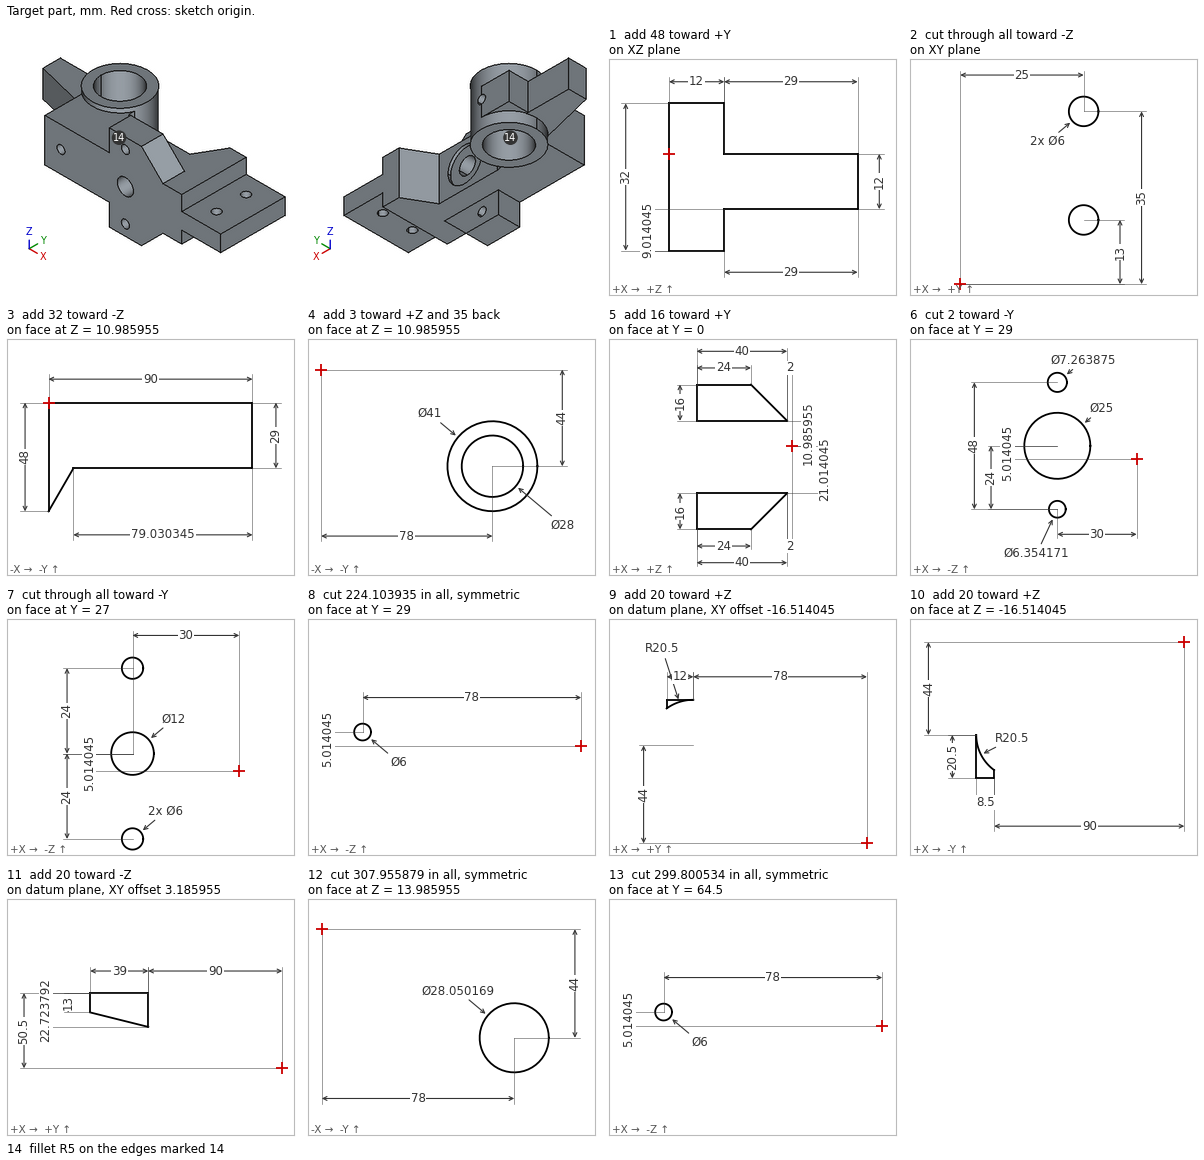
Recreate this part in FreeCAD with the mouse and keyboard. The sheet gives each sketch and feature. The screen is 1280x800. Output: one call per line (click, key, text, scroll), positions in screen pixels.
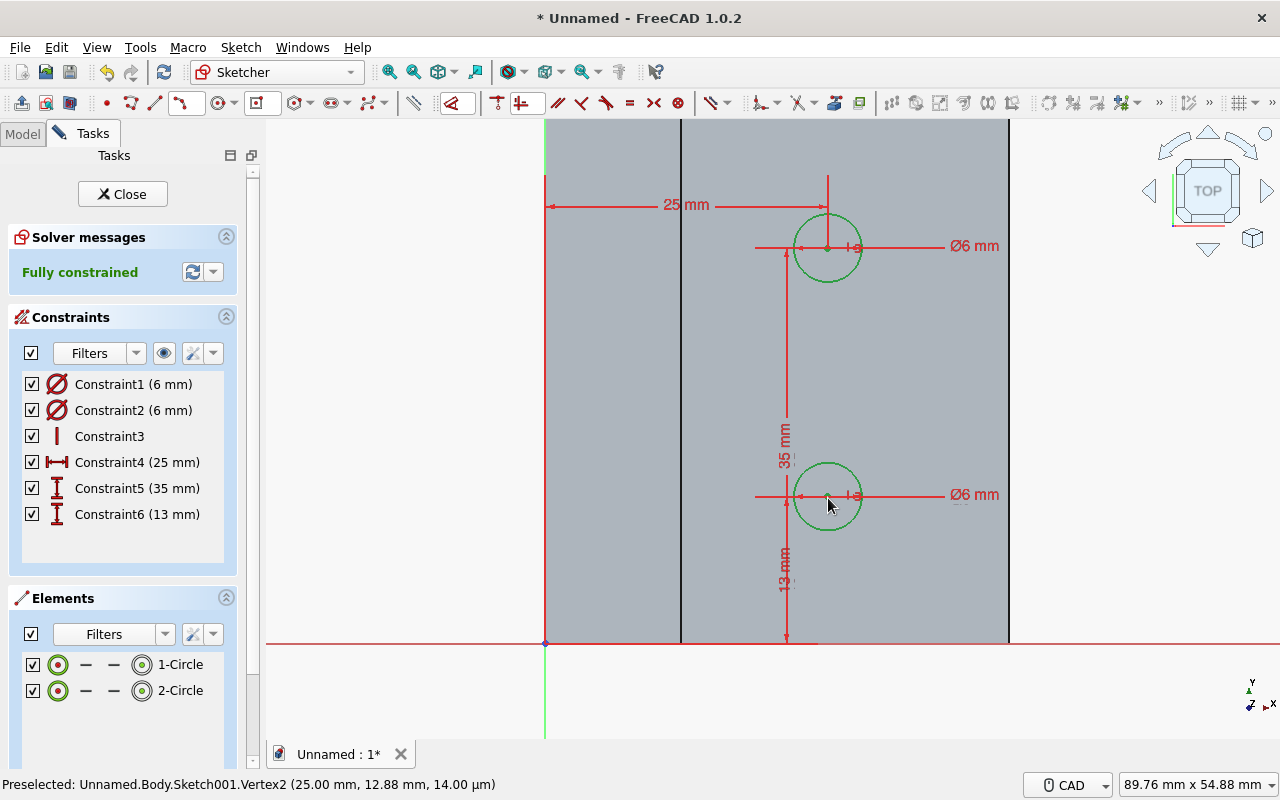
click(123, 194)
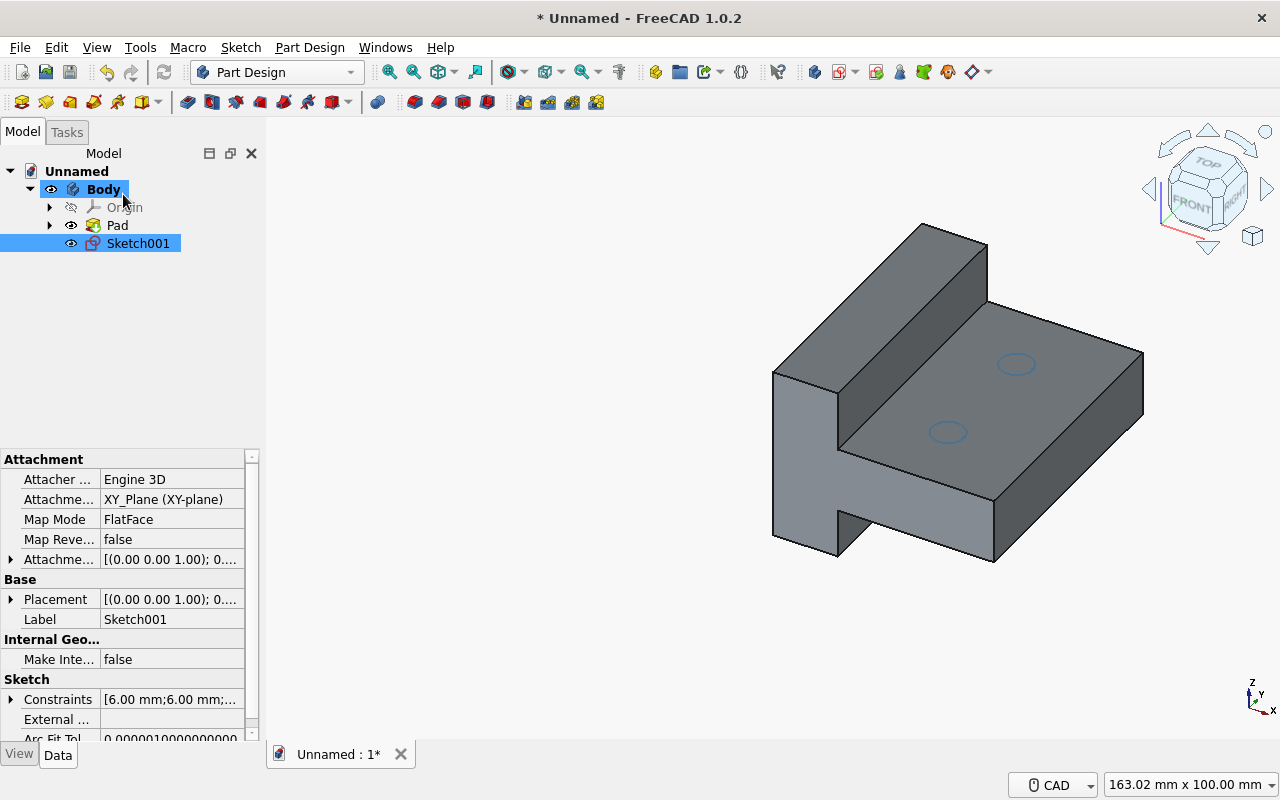
click(188, 102)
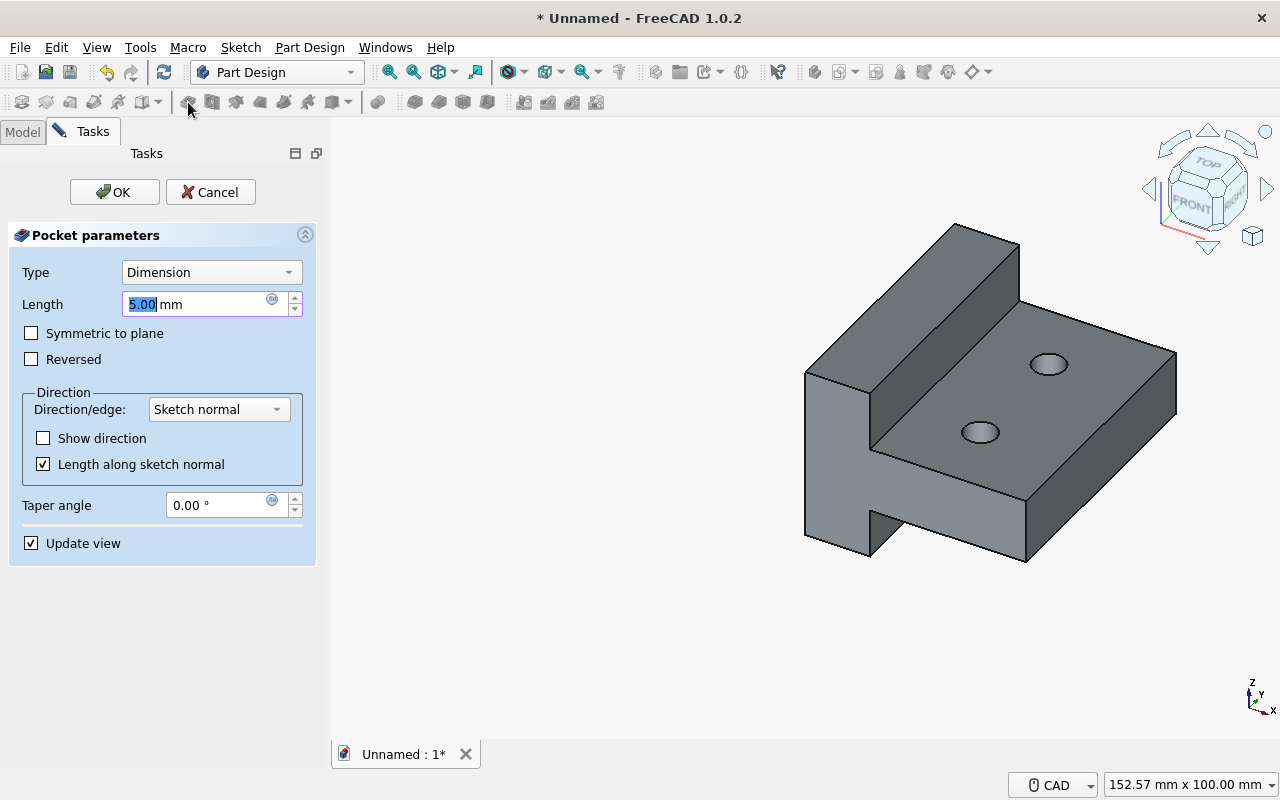
click(212, 272)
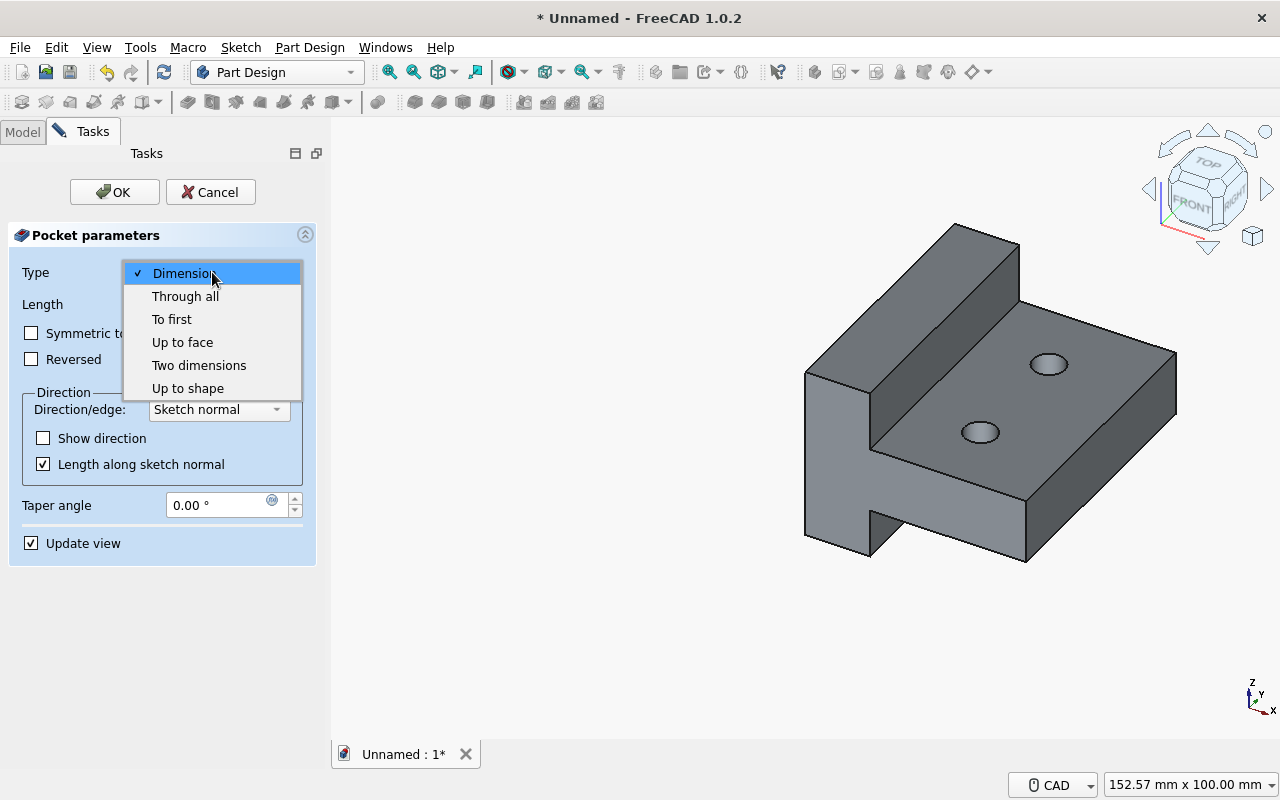
click(212, 296)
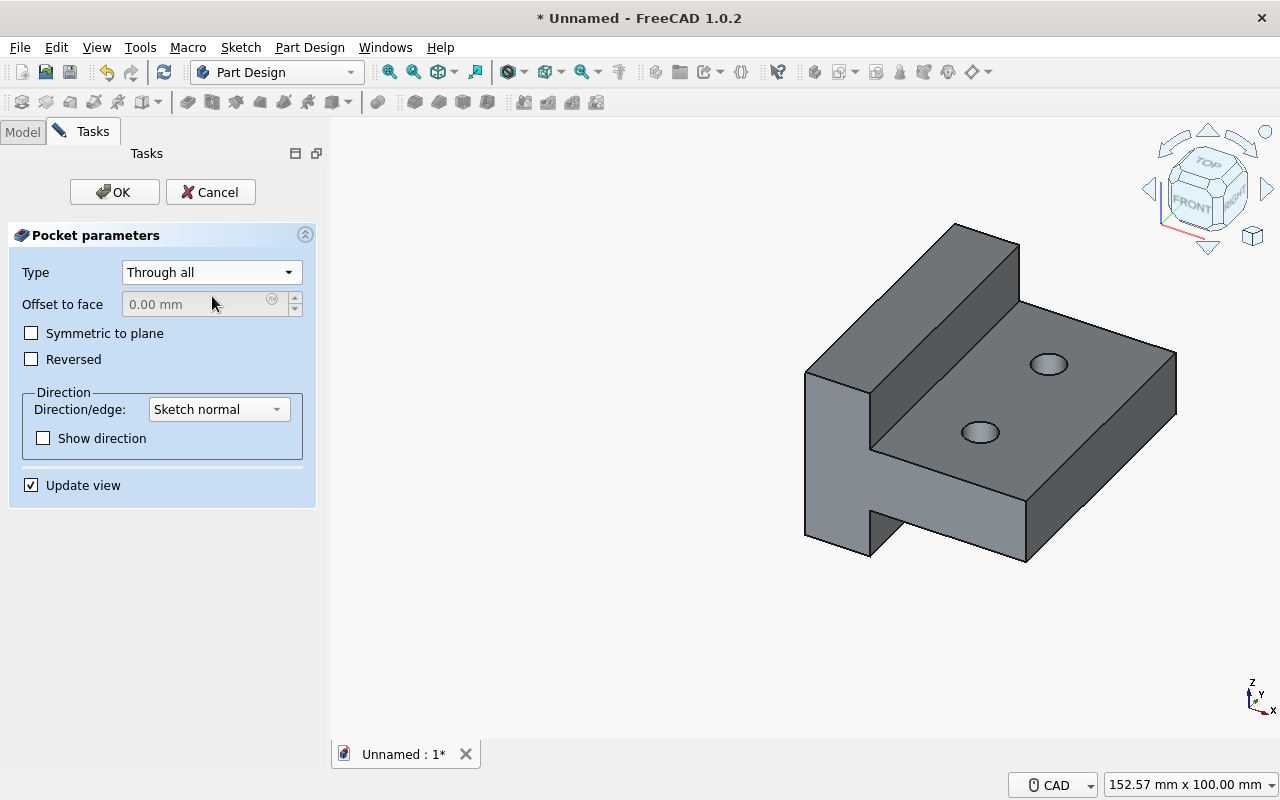
click(115, 192)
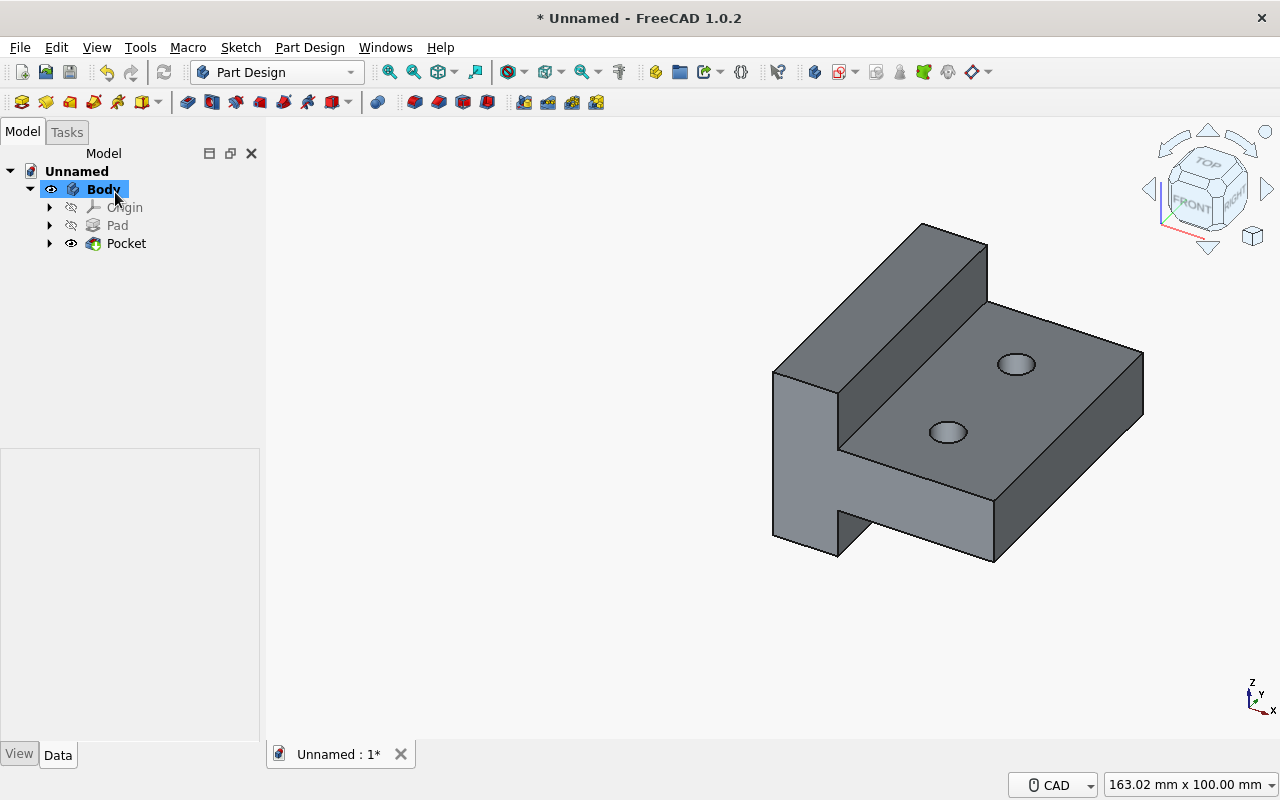
click(923, 265)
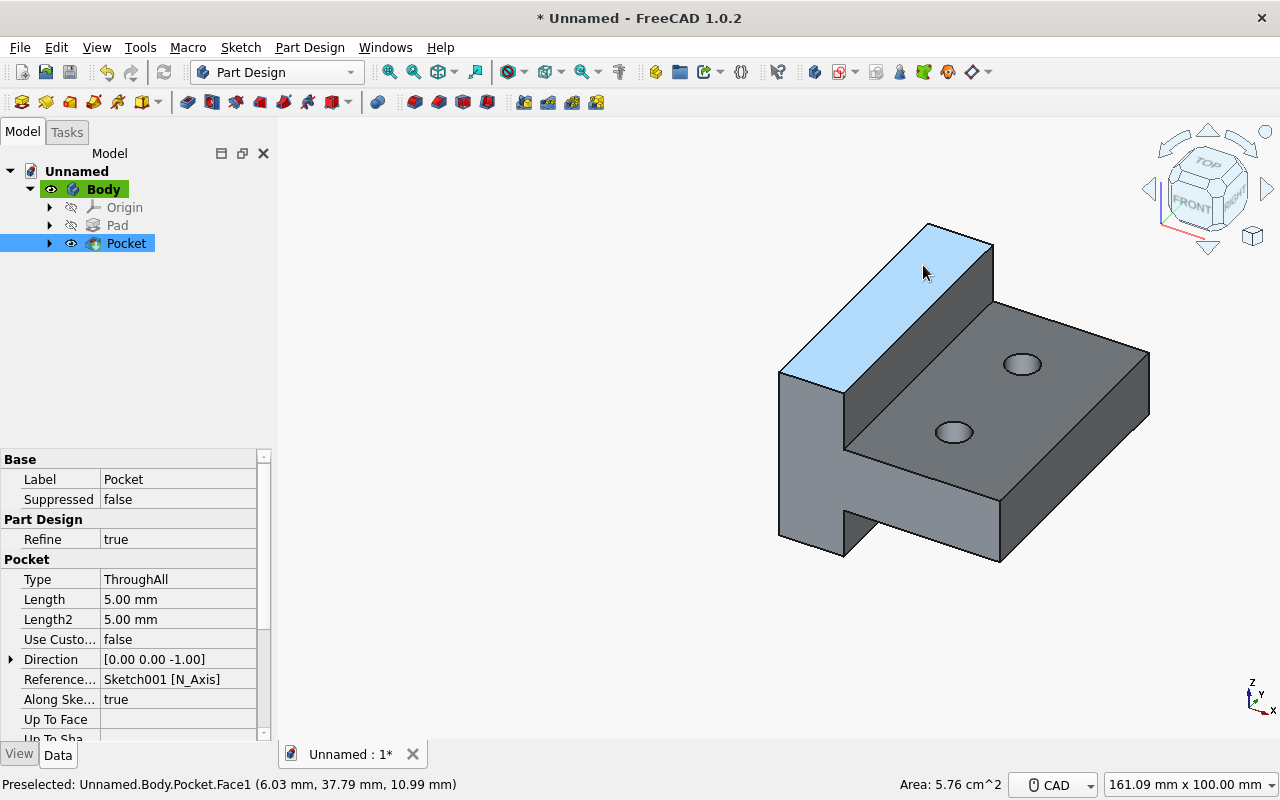
click(840, 72)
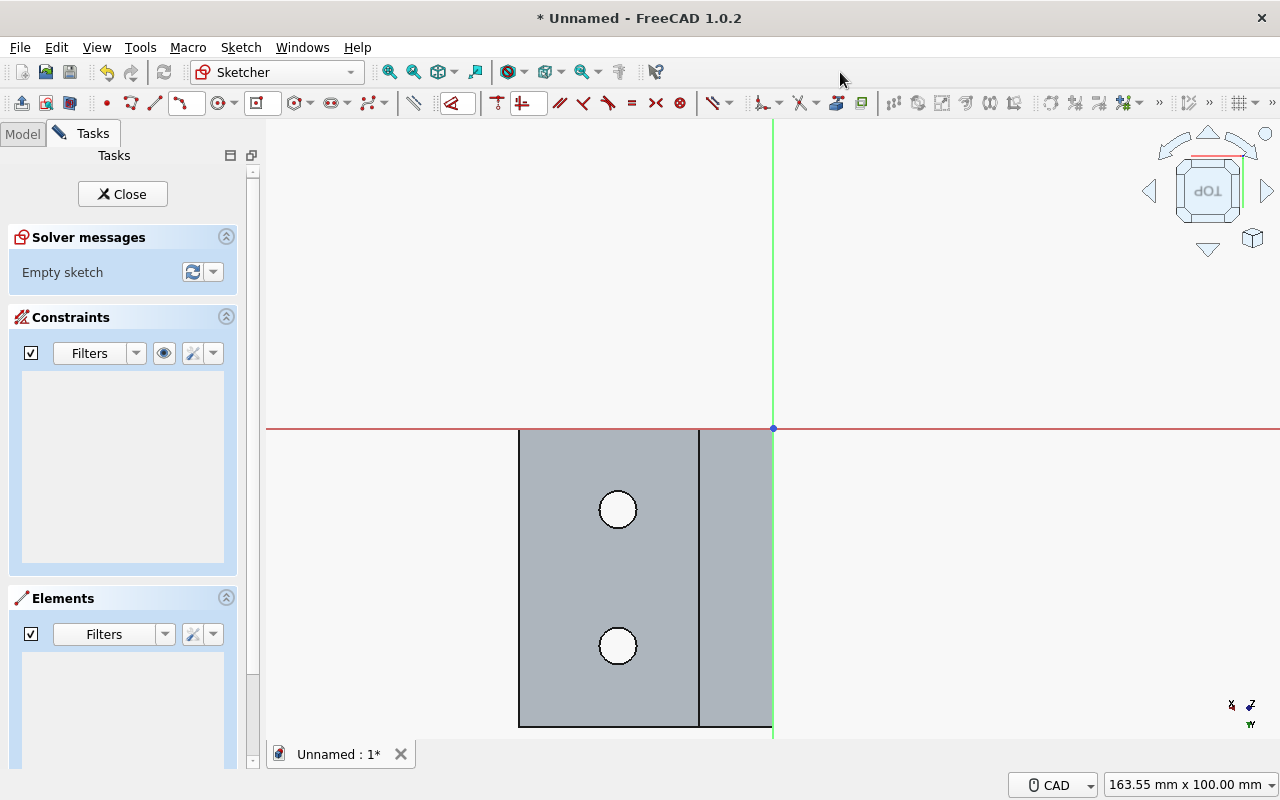
scroll(294, 147, down, 2)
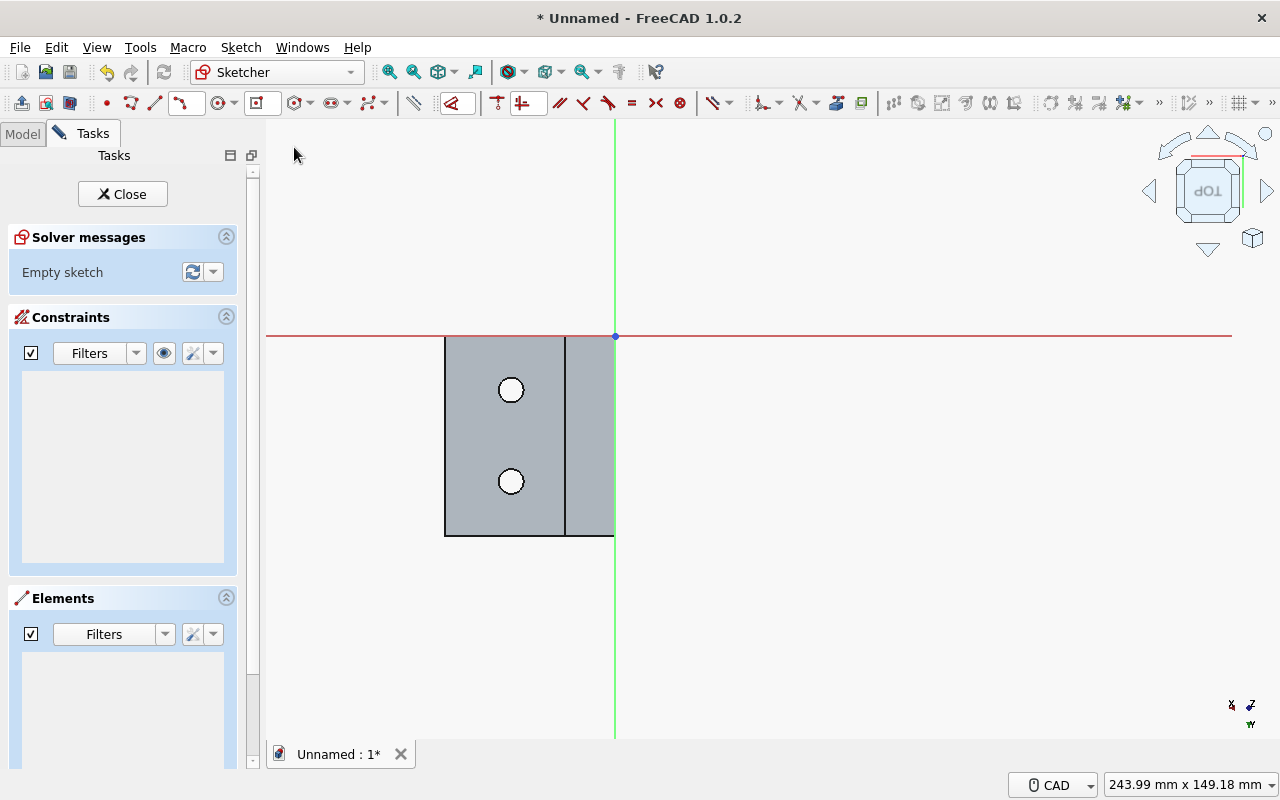
scroll(1001, 450, up, 2)